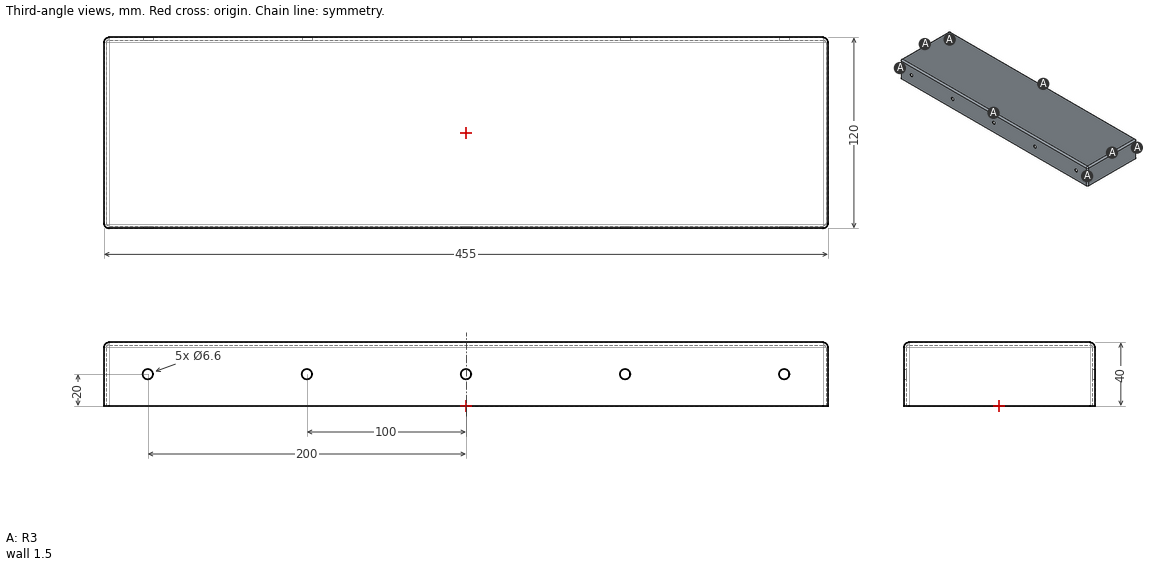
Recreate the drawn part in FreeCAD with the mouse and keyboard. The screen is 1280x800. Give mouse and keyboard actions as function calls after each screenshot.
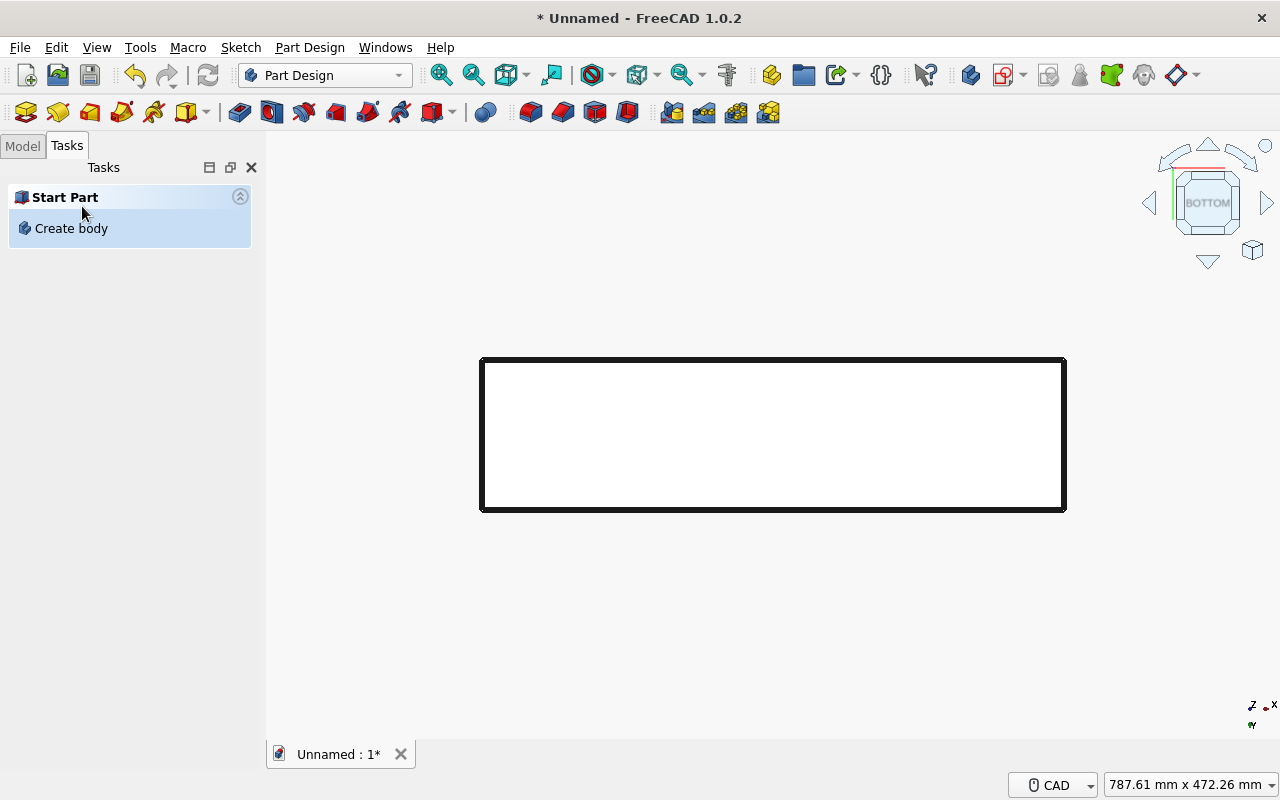
key(0)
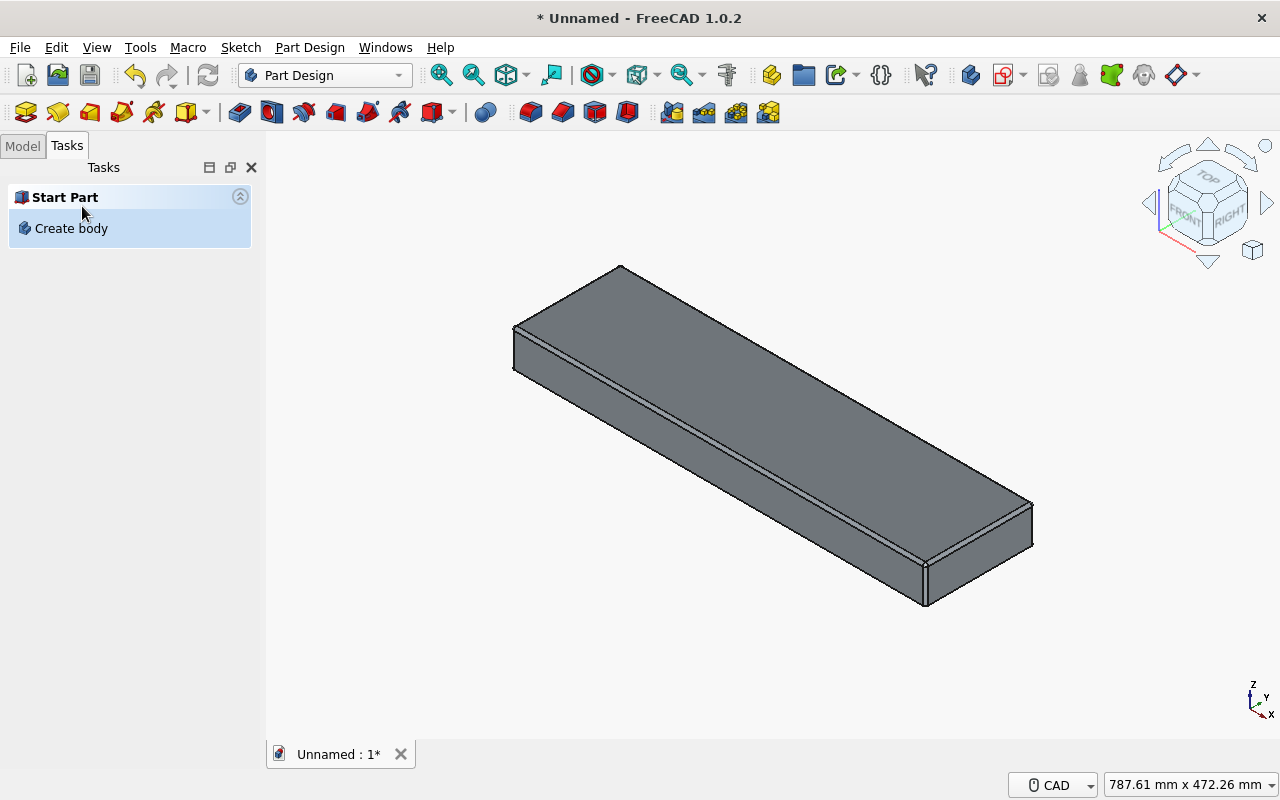
click(894, 568)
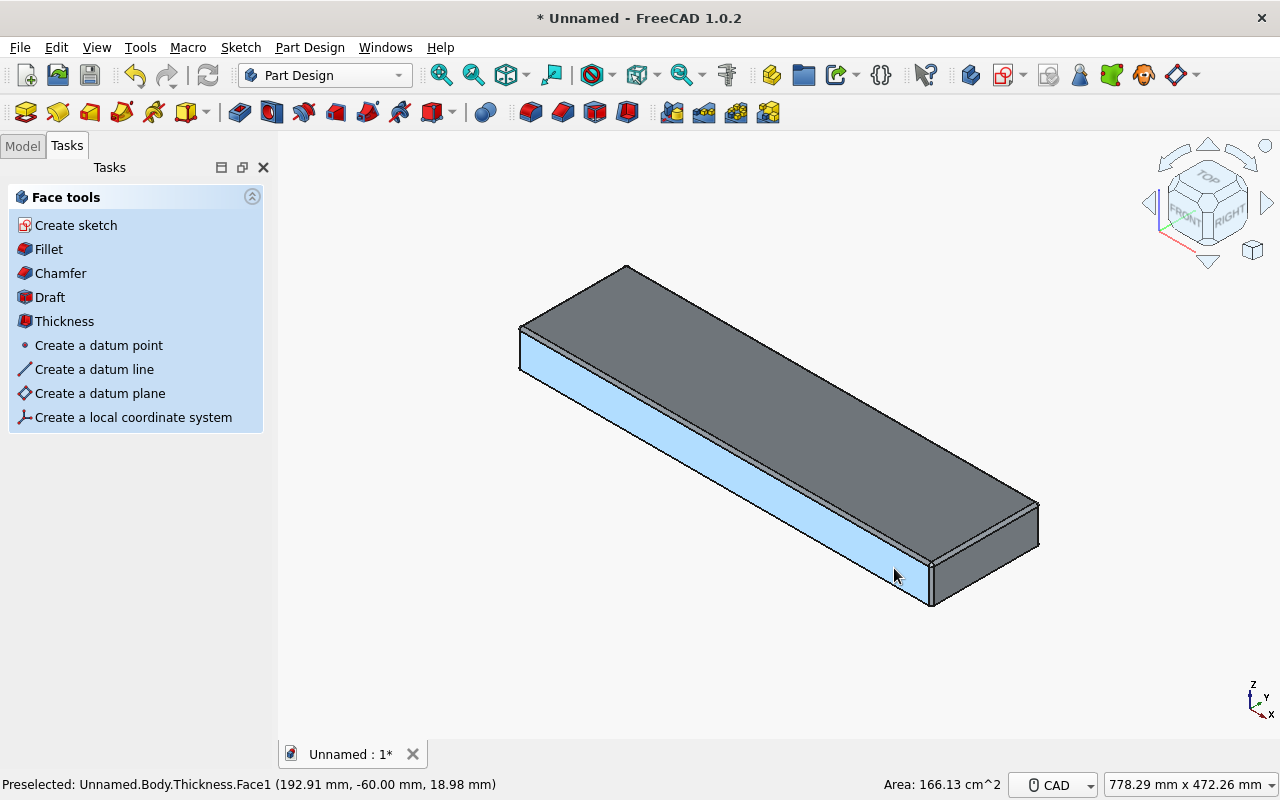
click(1004, 76)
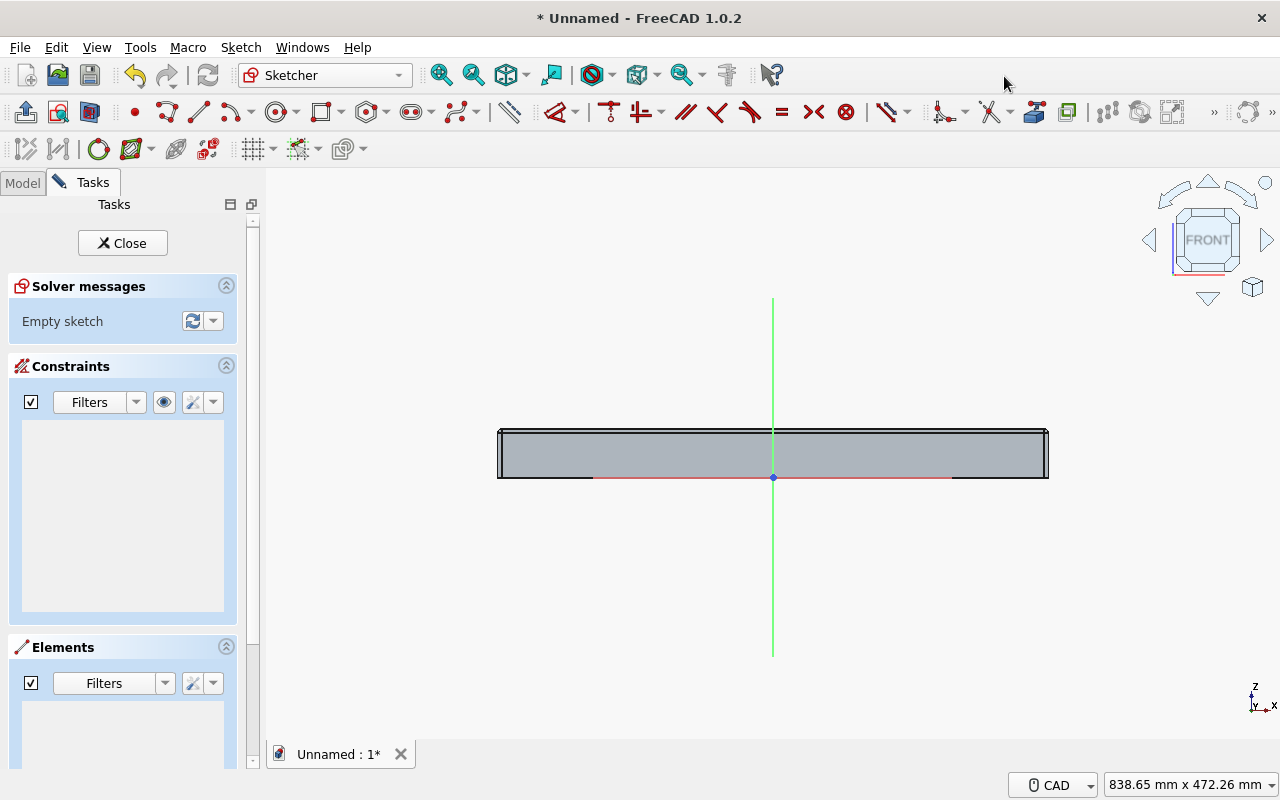
click(276, 112)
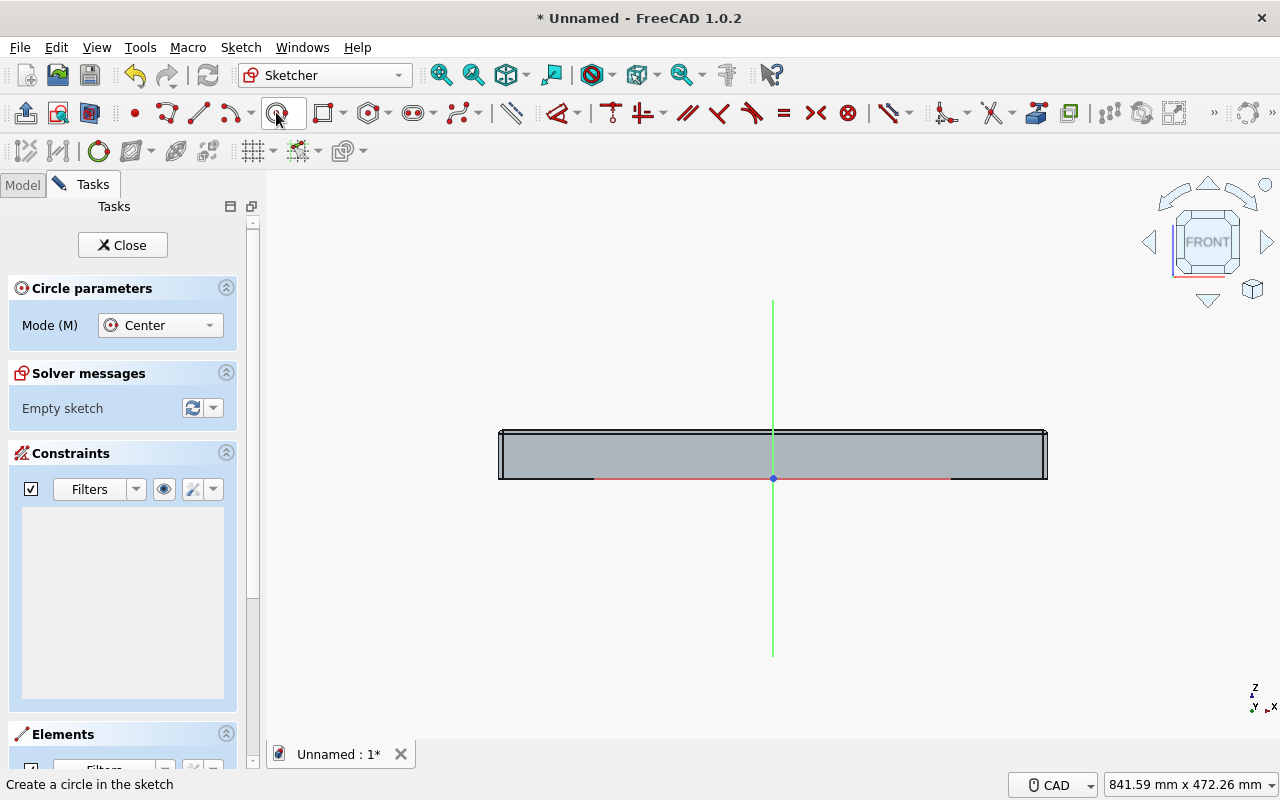
scroll(532, 454, up, 9)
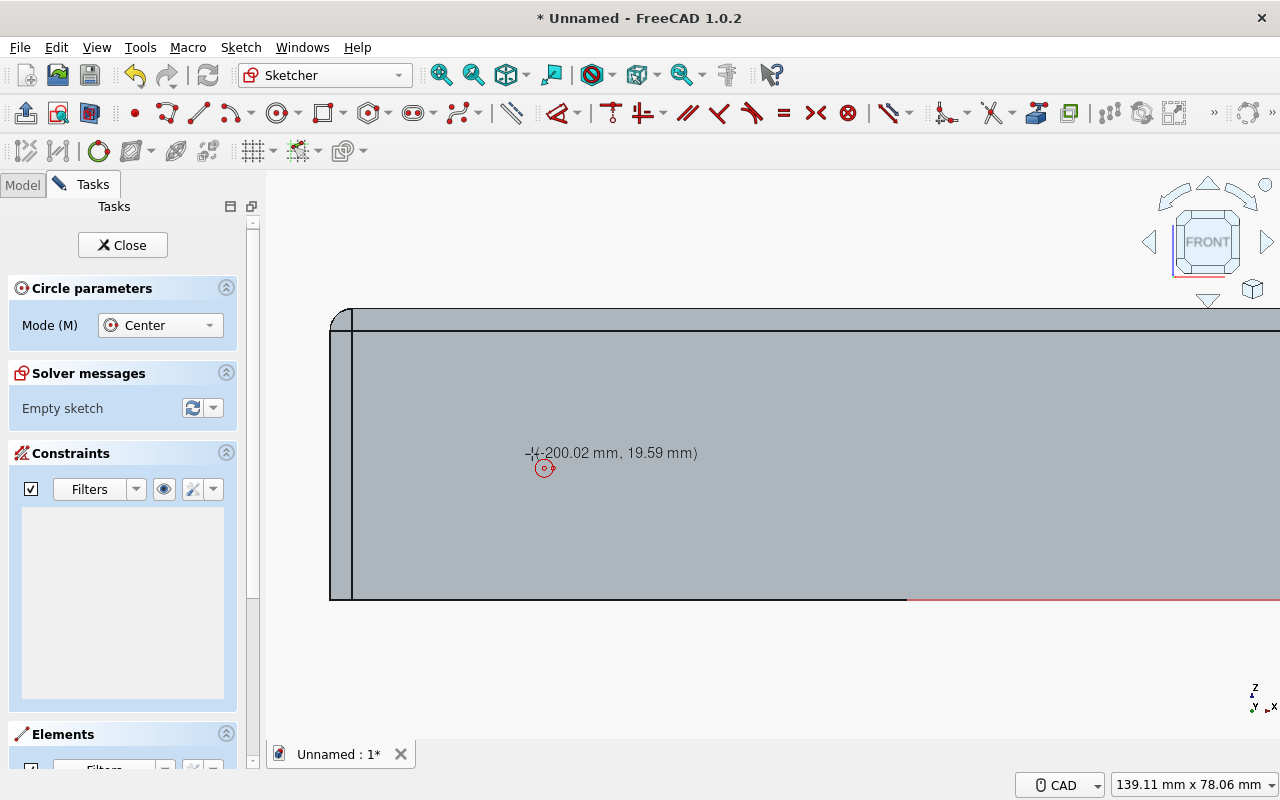
scroll(380, 439, down, 8)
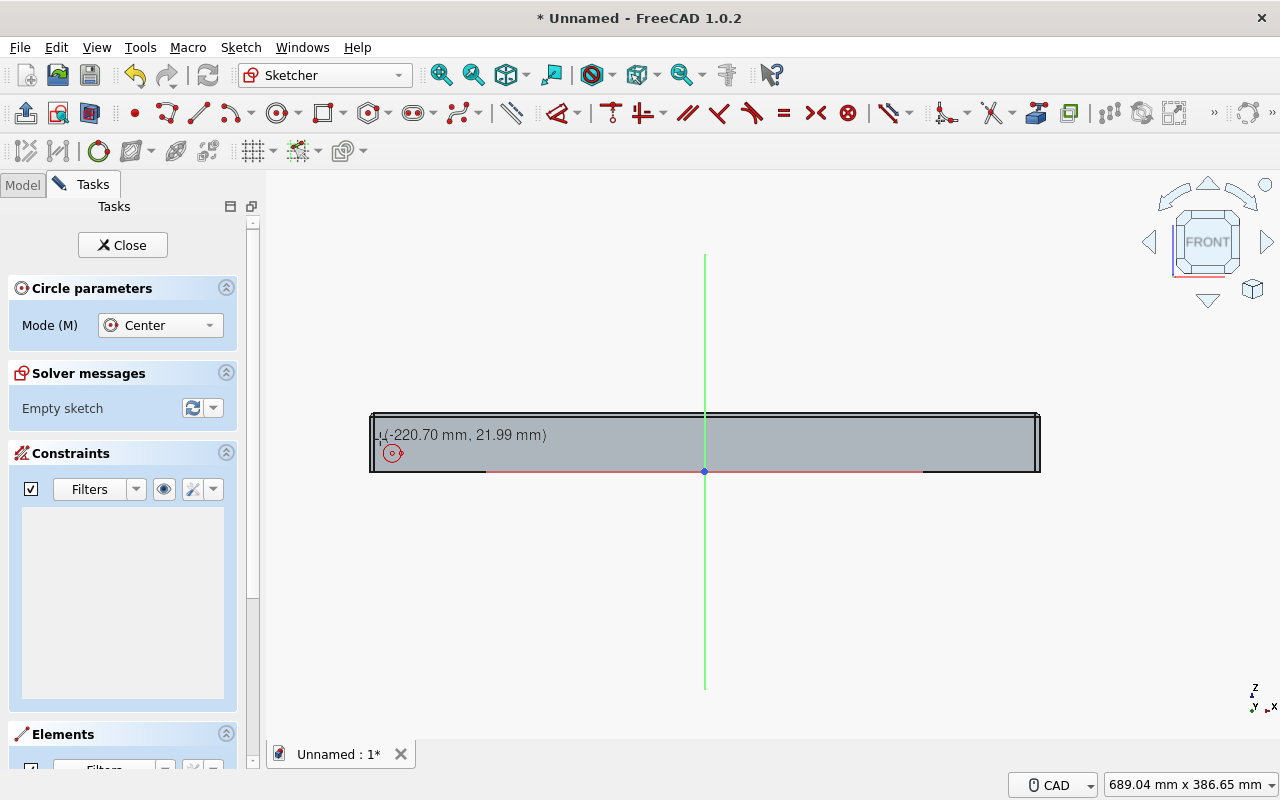
click(411, 443)
move(414, 439)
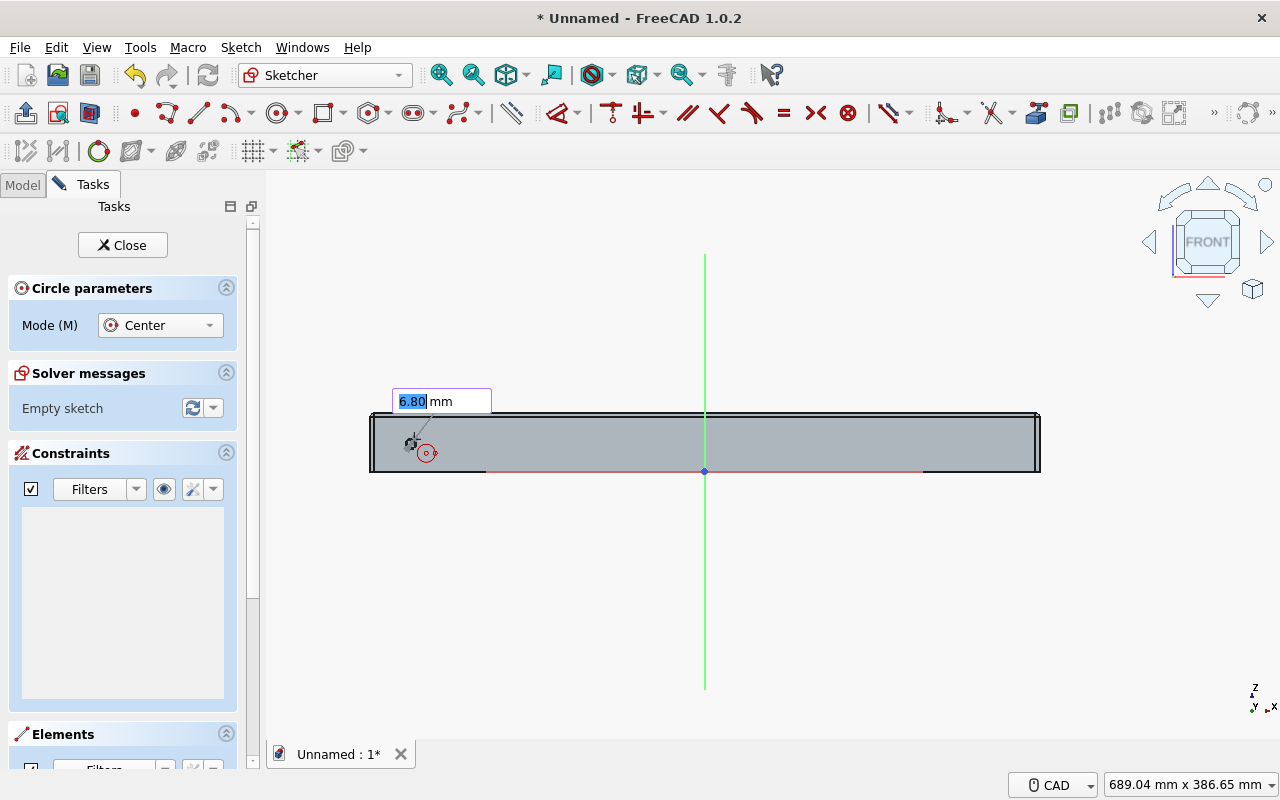
text(6.6)
key(Return)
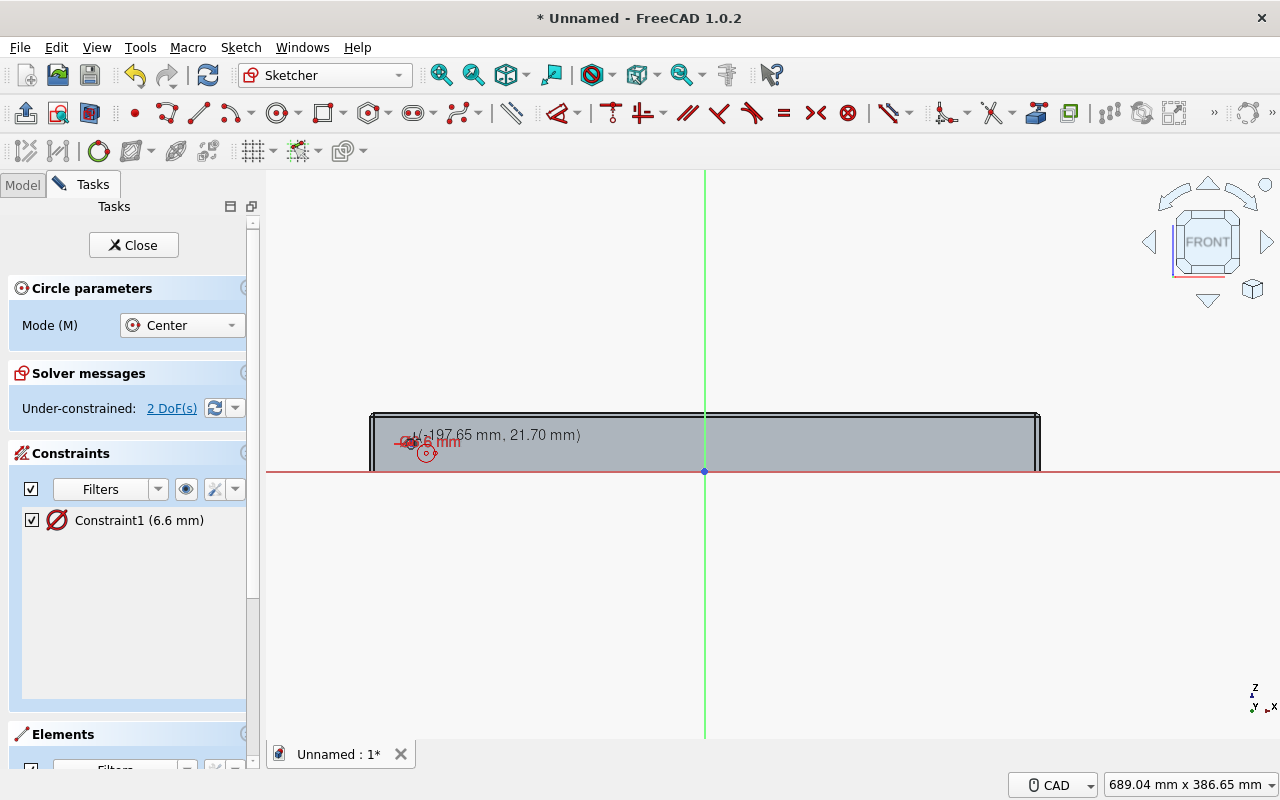
scroll(558, 443, up, 8)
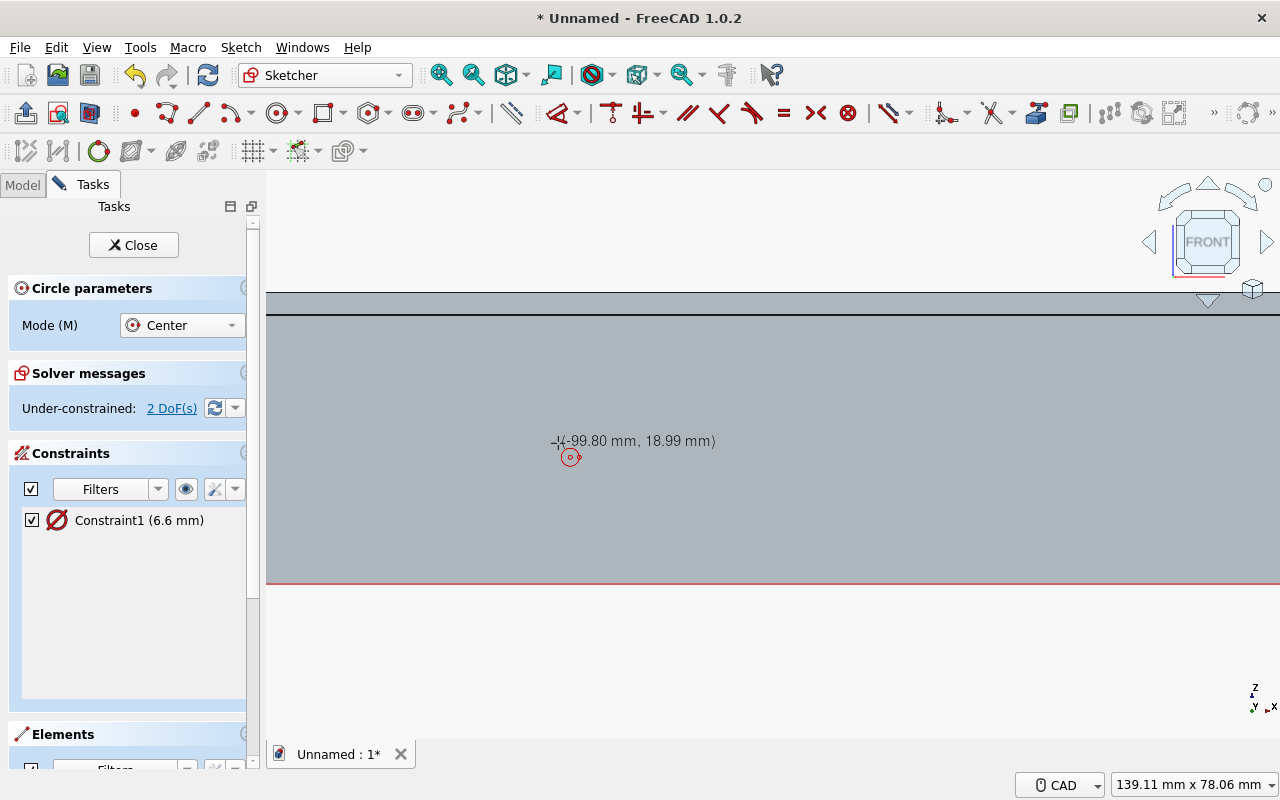
scroll(558, 443, down, 8)